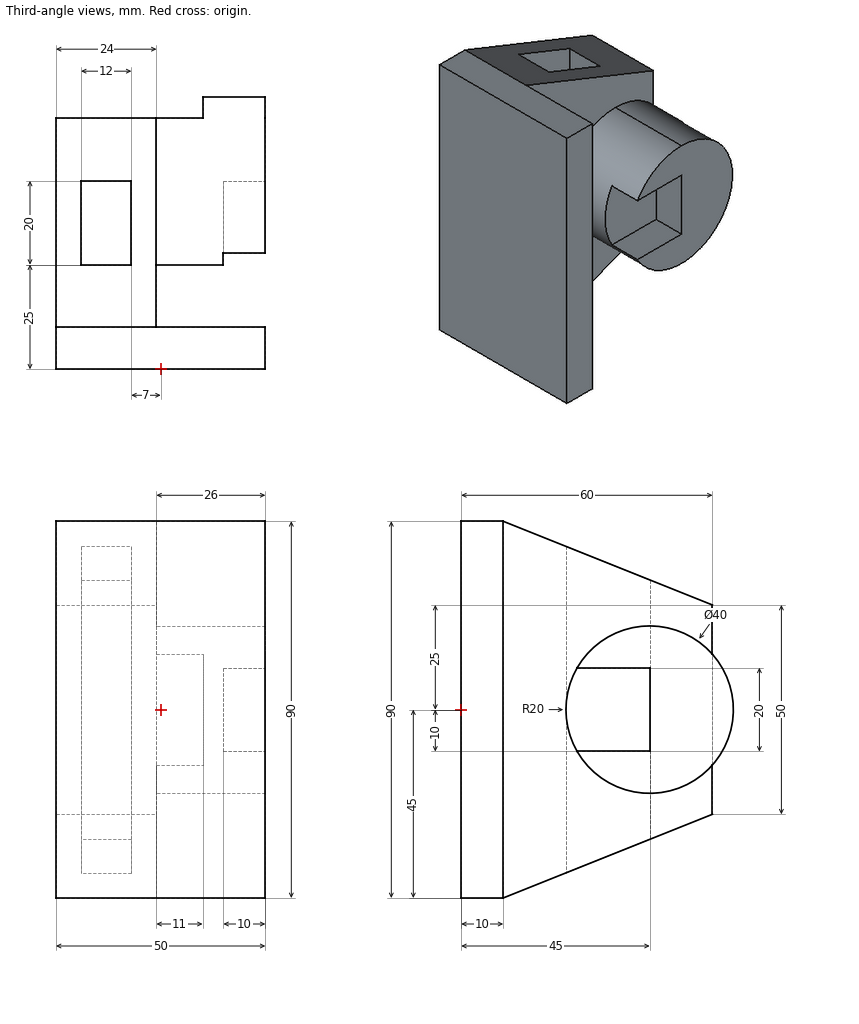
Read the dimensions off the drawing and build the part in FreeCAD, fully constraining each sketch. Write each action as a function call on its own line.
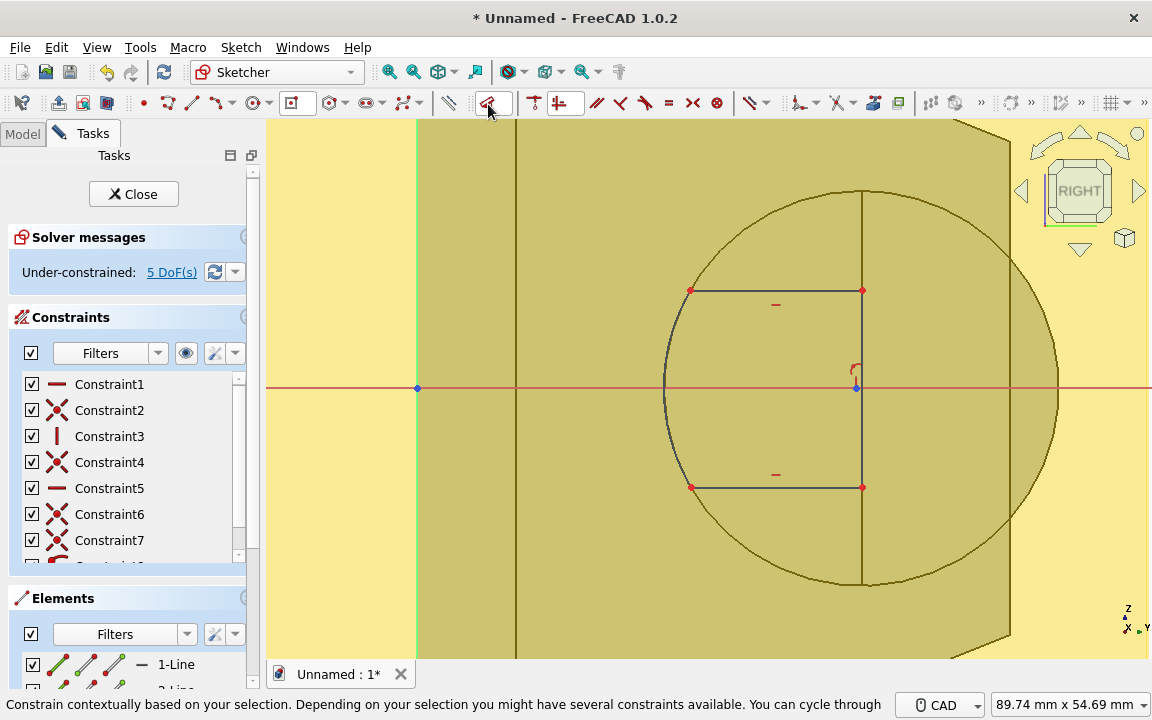
click(668, 349)
click(637, 342)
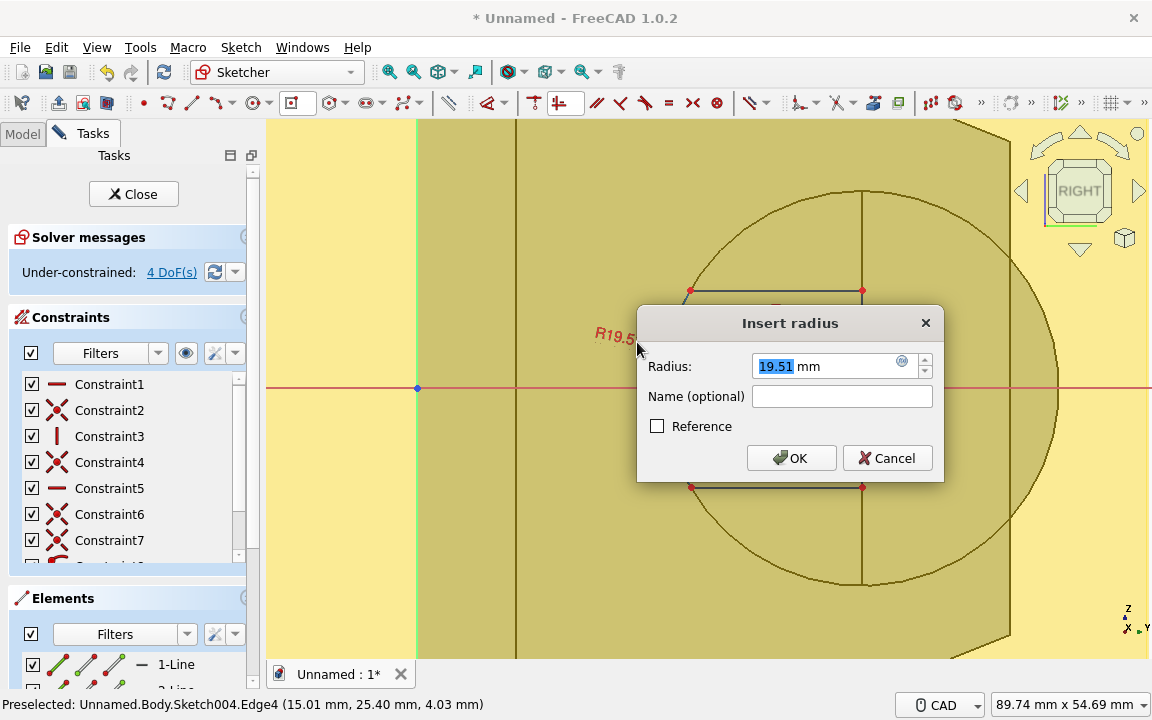
text(20)
key(Return)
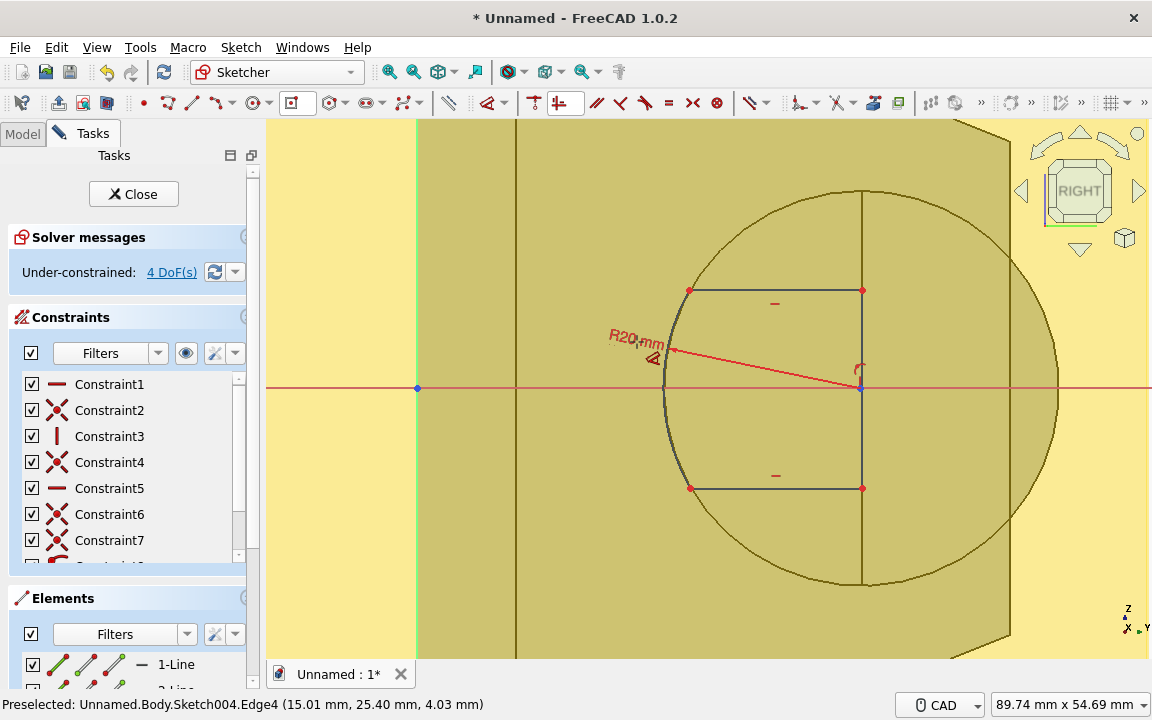
click(862, 429)
click(896, 344)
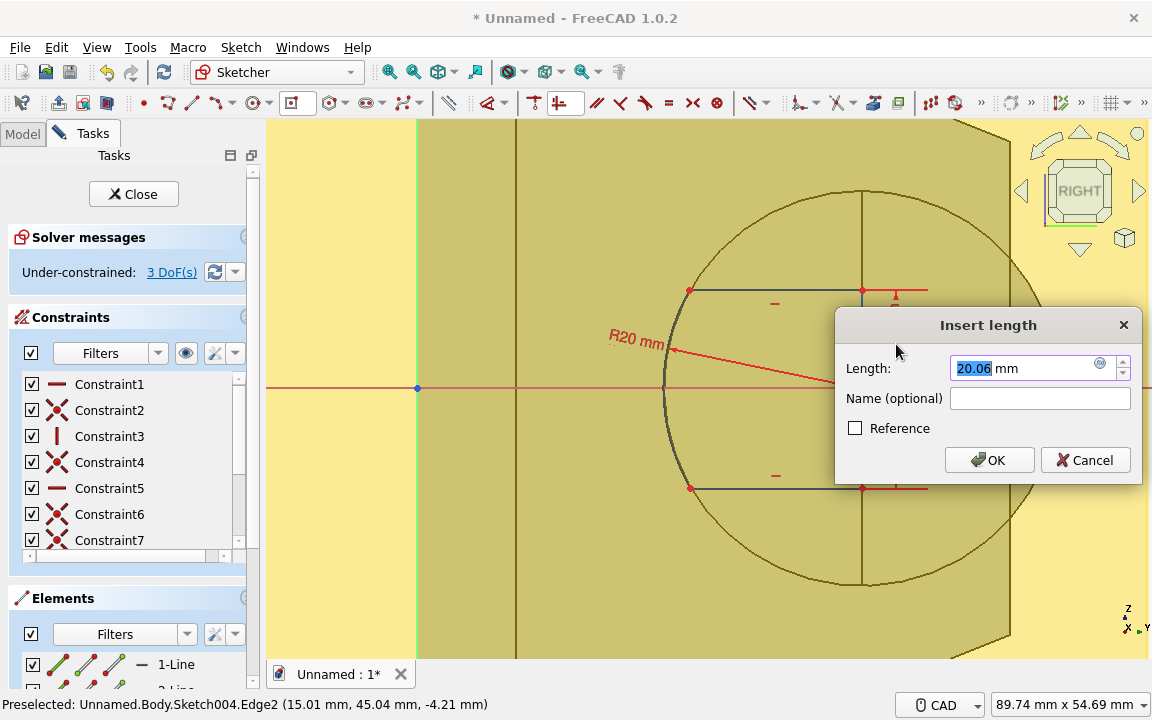
text(20)
key(Return)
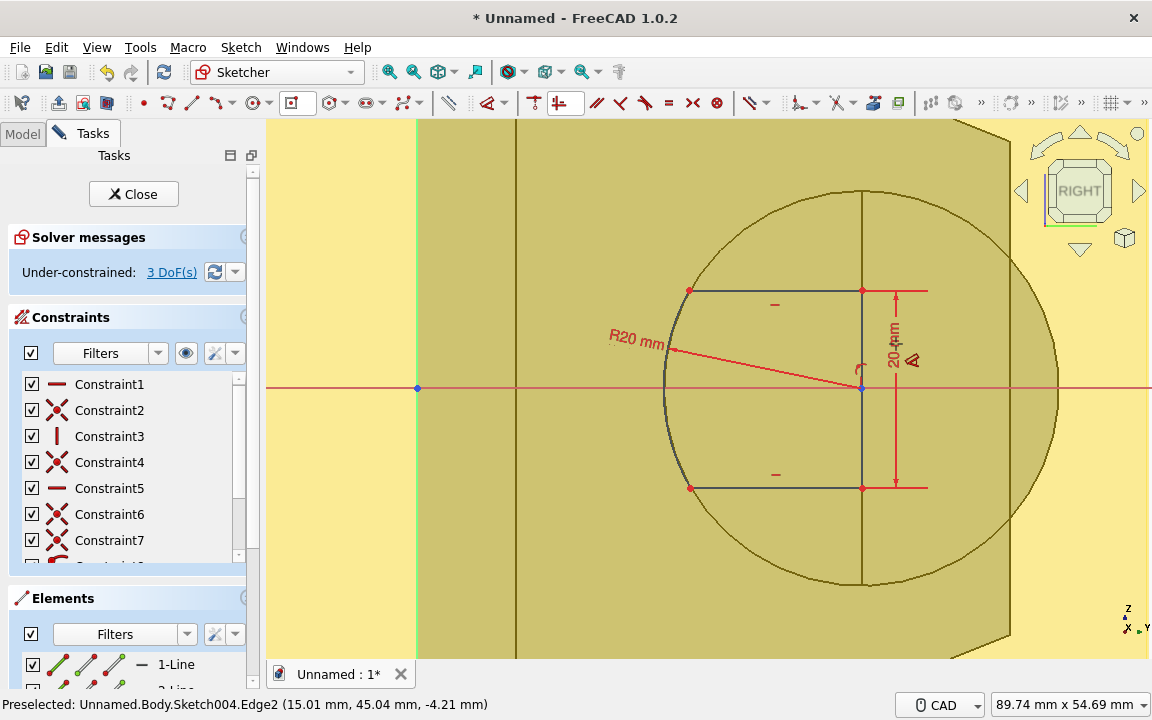
click(691, 488)
click(383, 438)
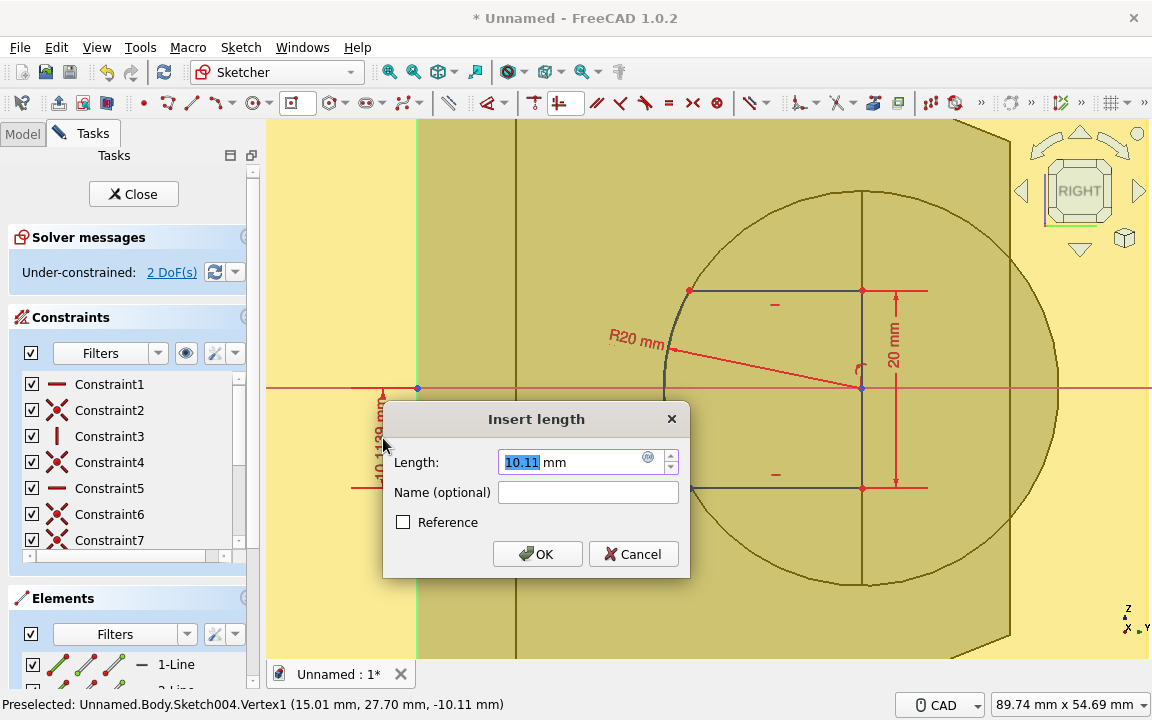
text(10)
key(Return)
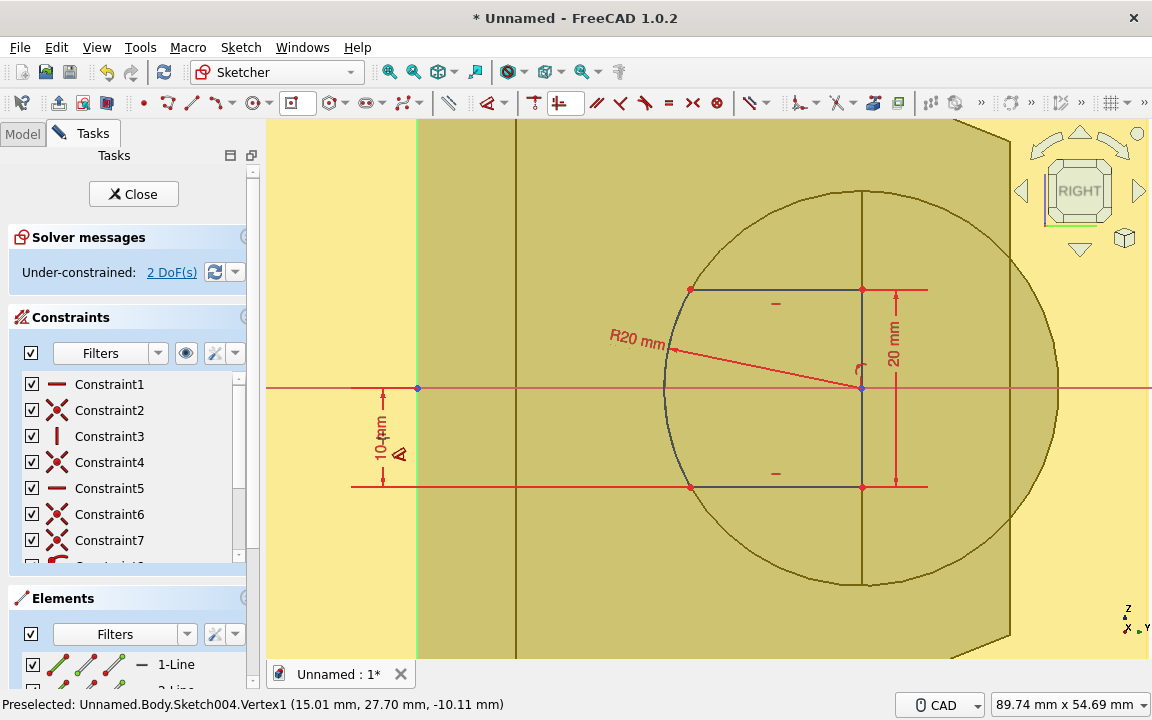
click(862, 487)
click(640, 521)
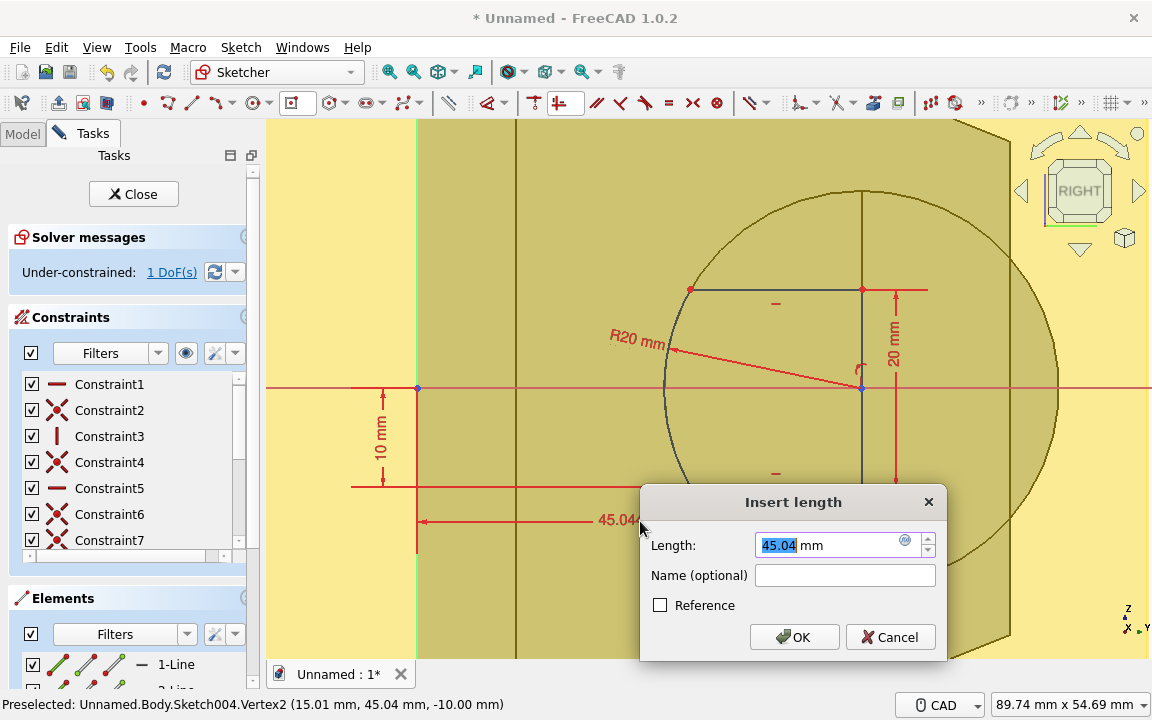
text(45)
key(Return)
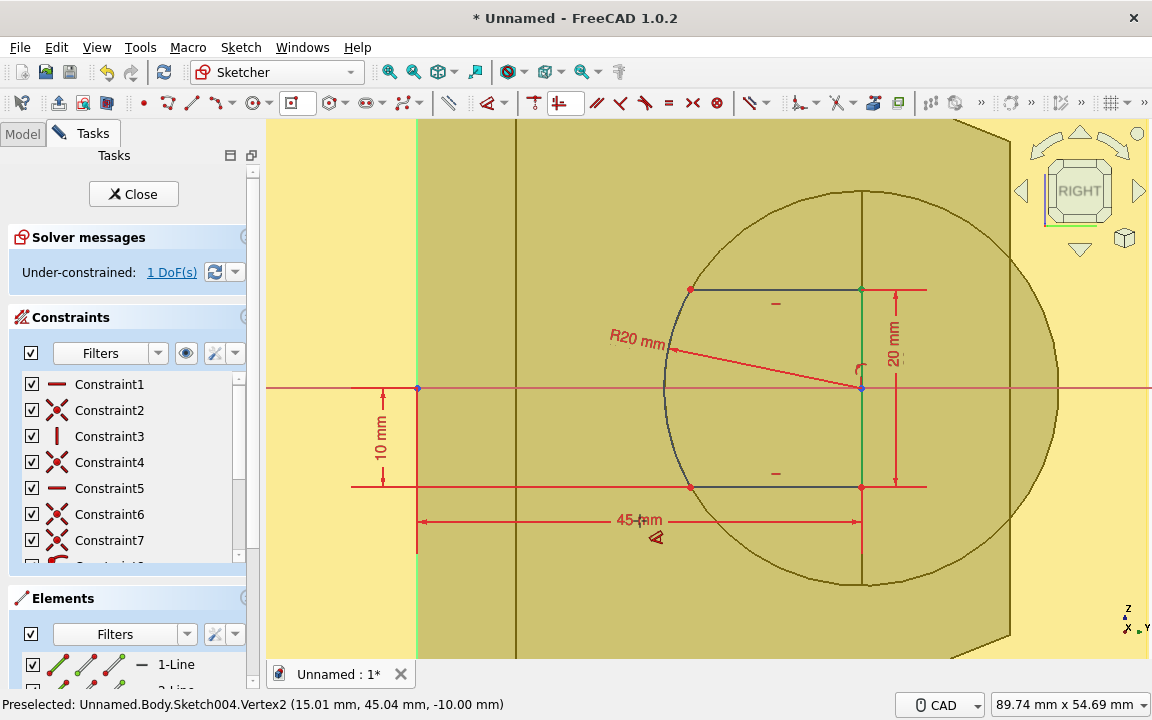
click(862, 388)
click(640, 422)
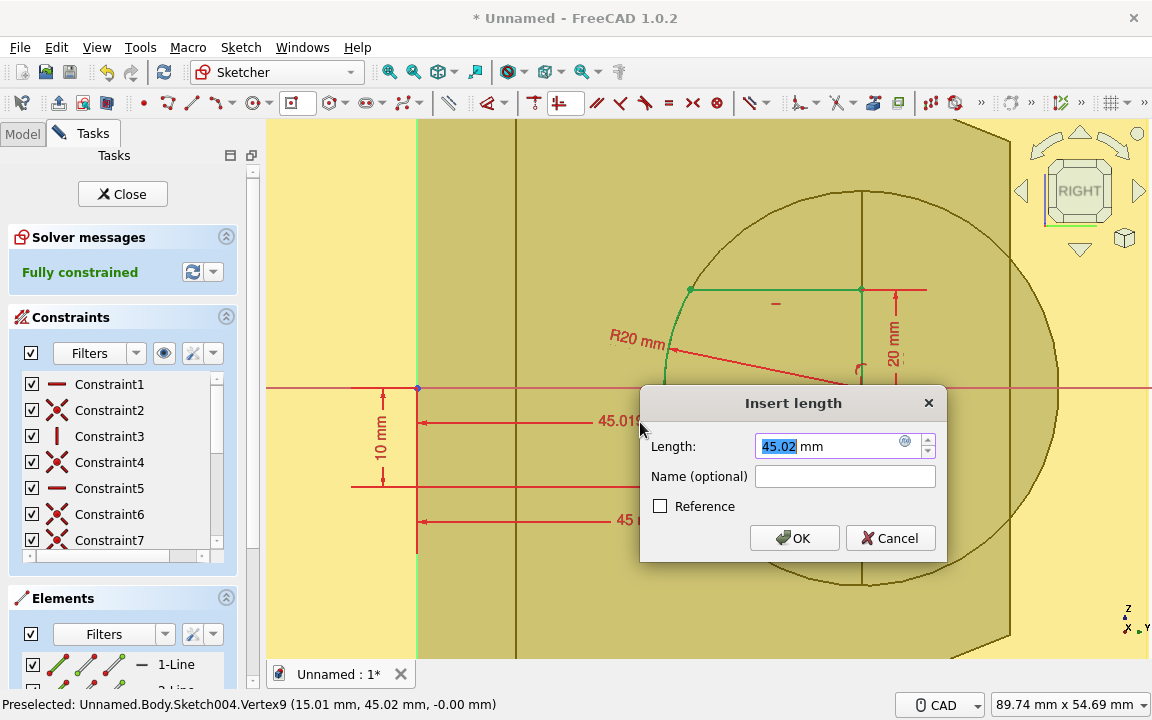
text(45)
key(Return)
key(Escape)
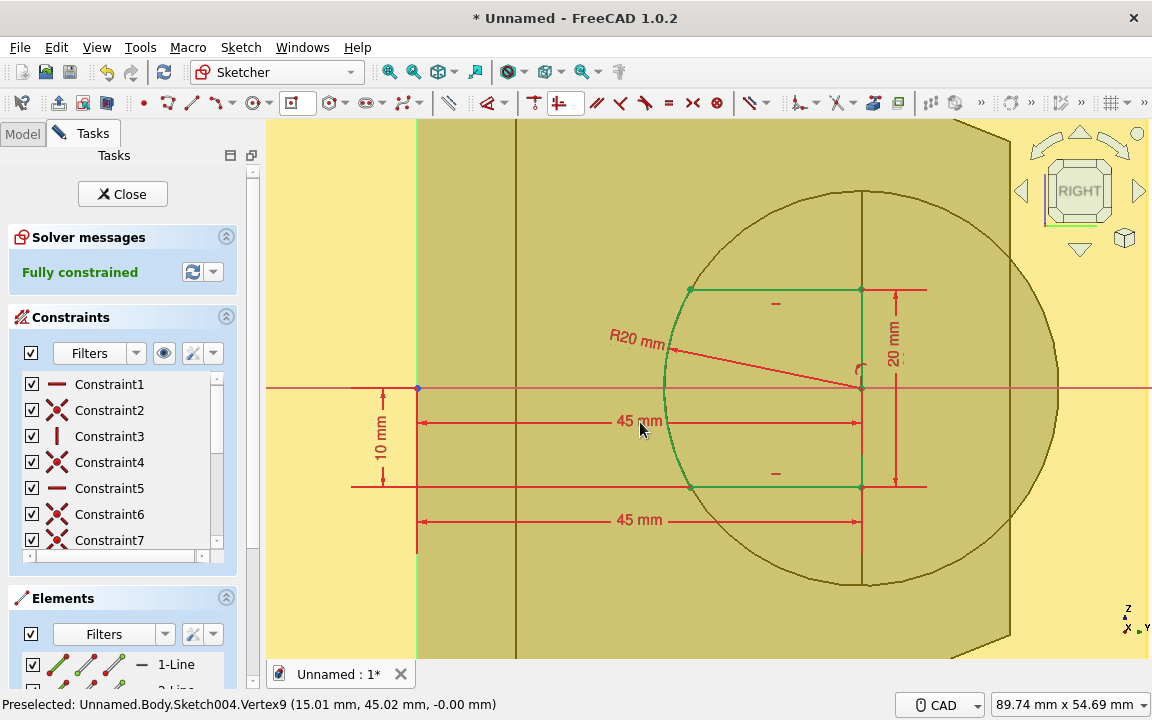
click(123, 194)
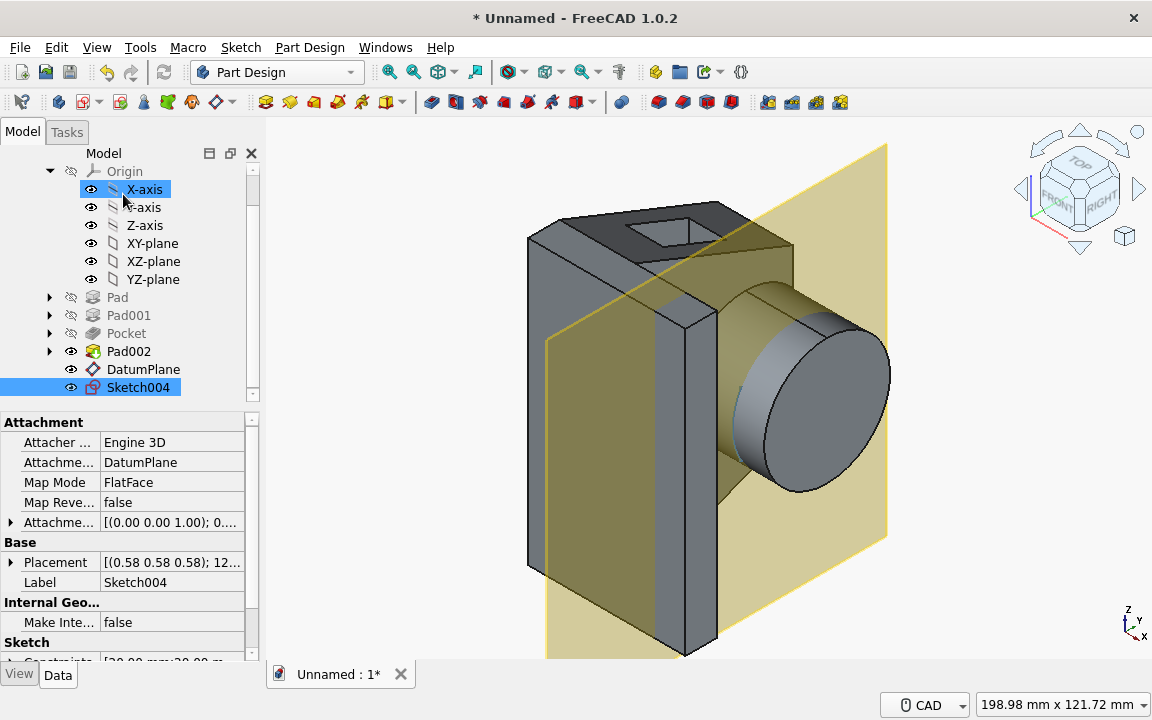
click(432, 102)